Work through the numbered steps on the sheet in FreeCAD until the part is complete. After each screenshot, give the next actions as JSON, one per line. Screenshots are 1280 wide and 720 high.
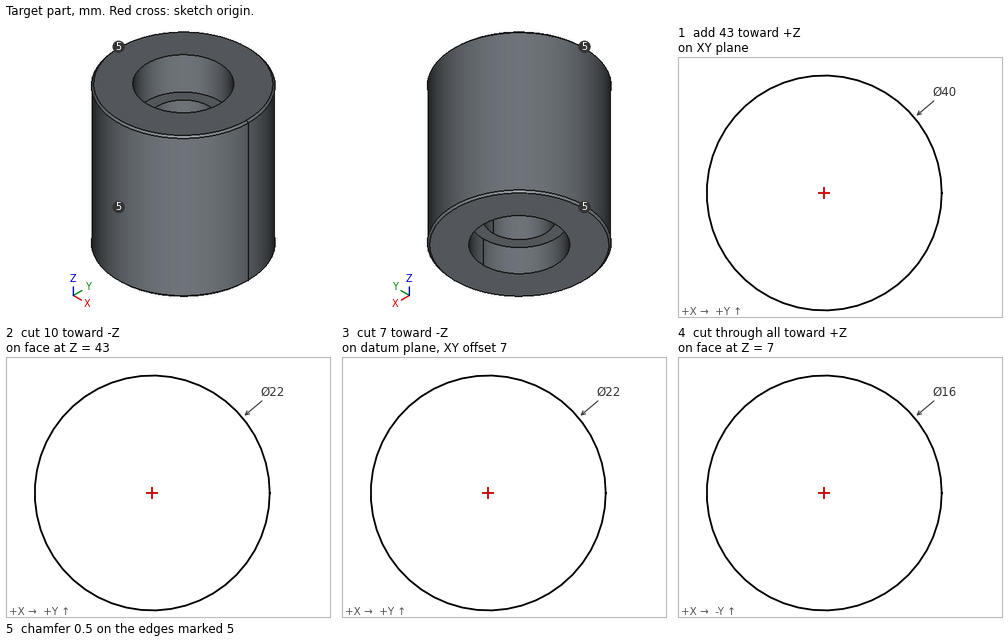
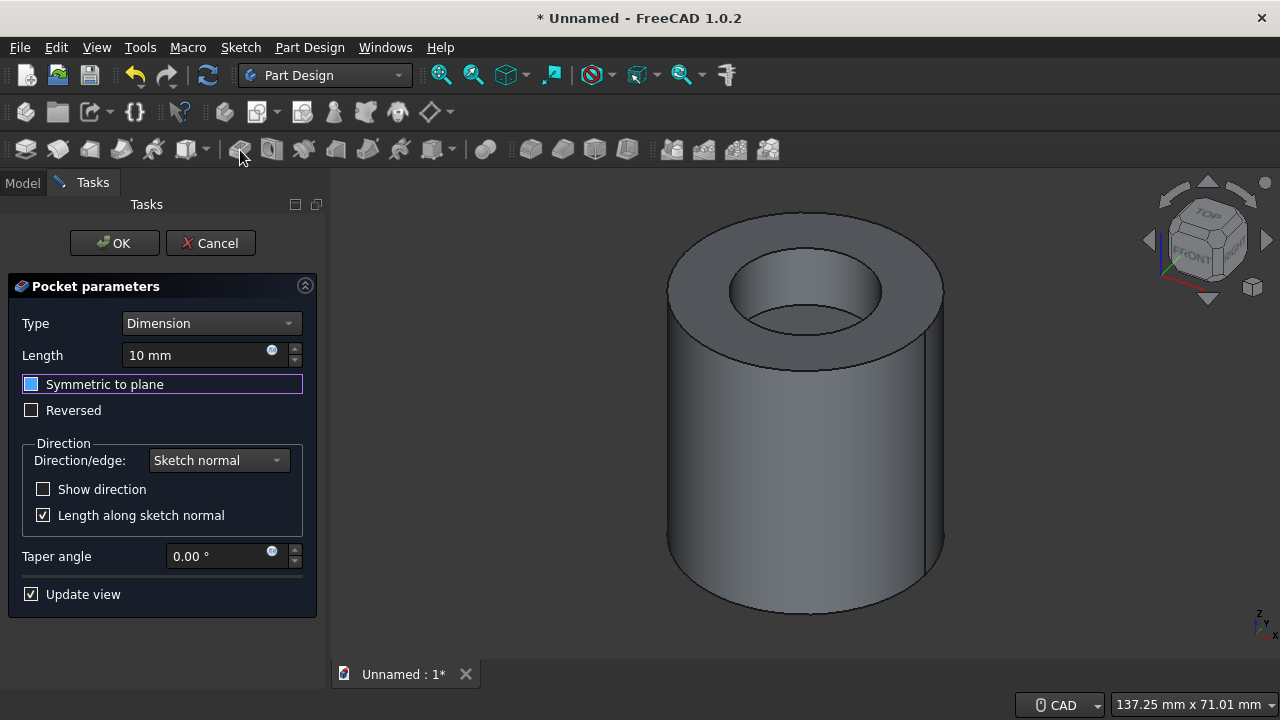
{"action": "left_click", "coordinate": [115, 243]}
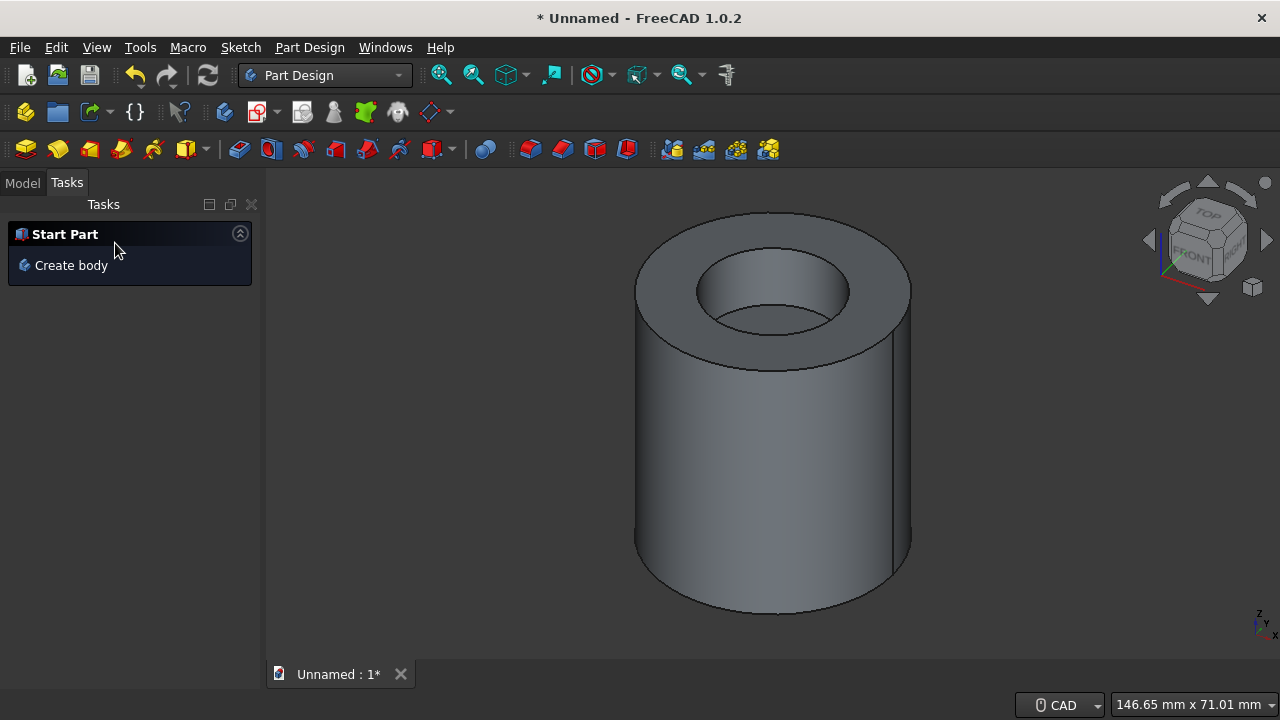
{"action": "left_click", "coordinate": [23, 182]}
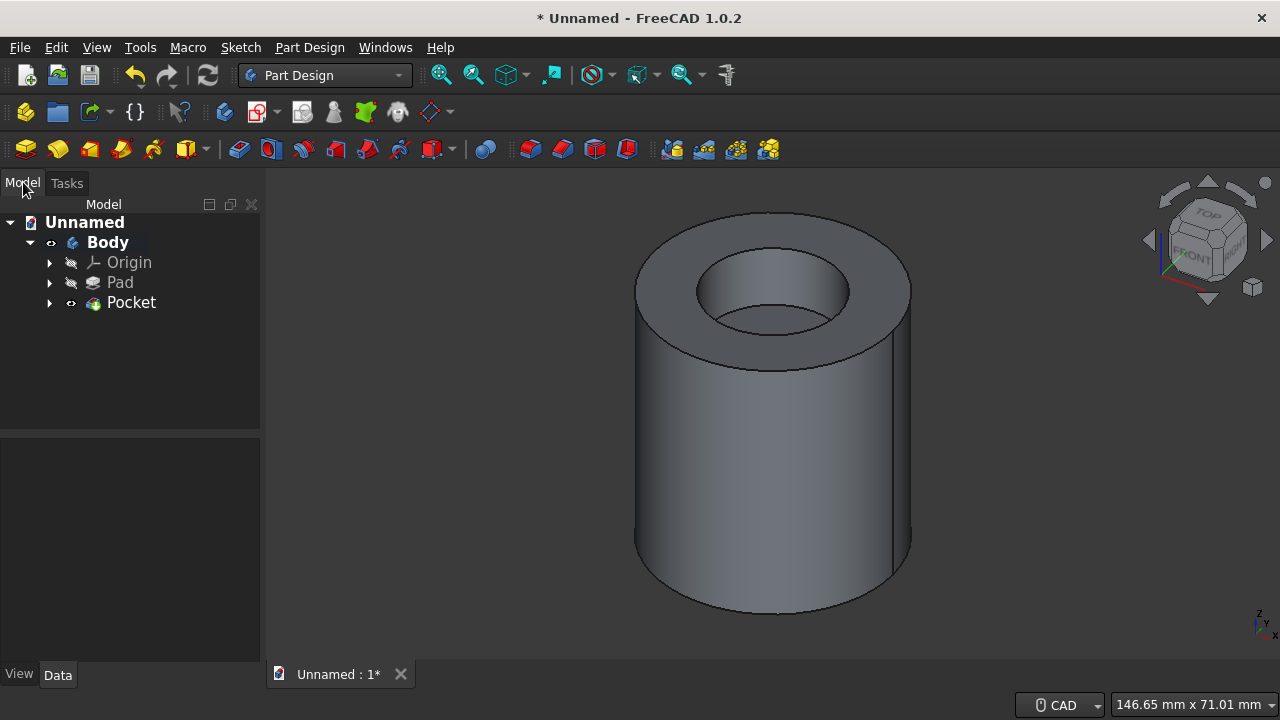
{"action": "left_click", "coordinate": [50, 263]}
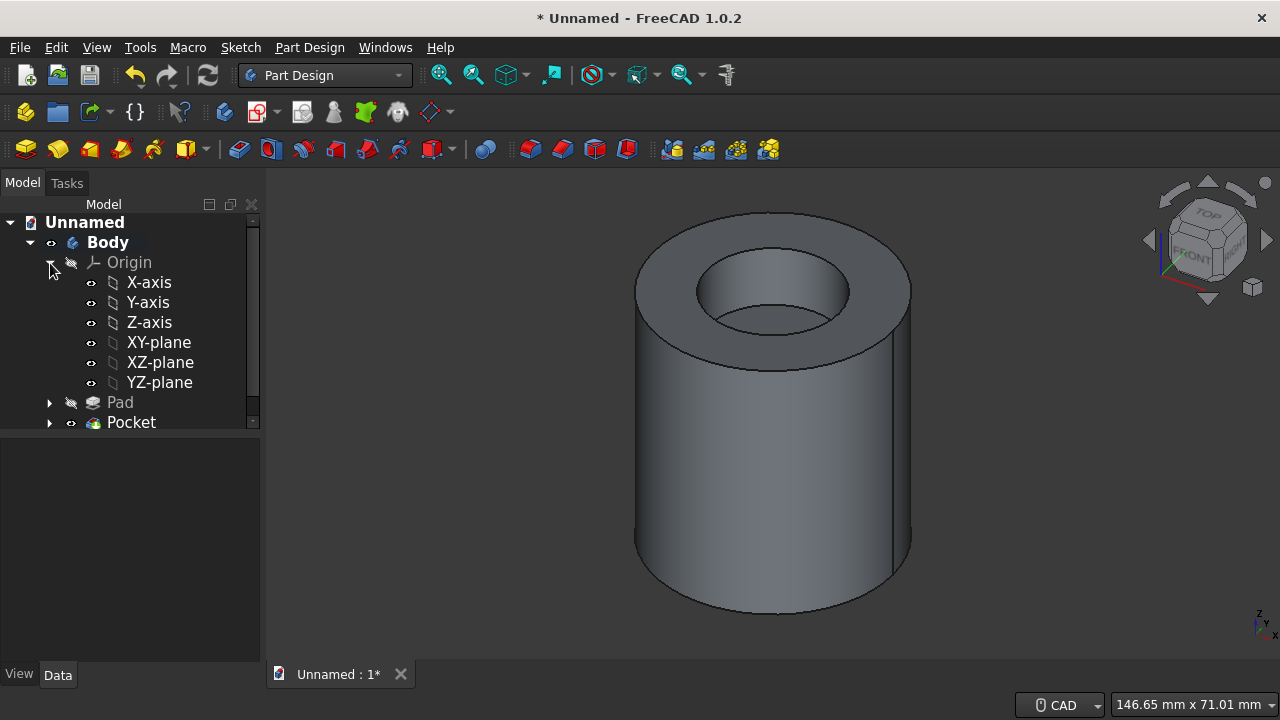
{"action": "left_click", "coordinate": [136, 343]}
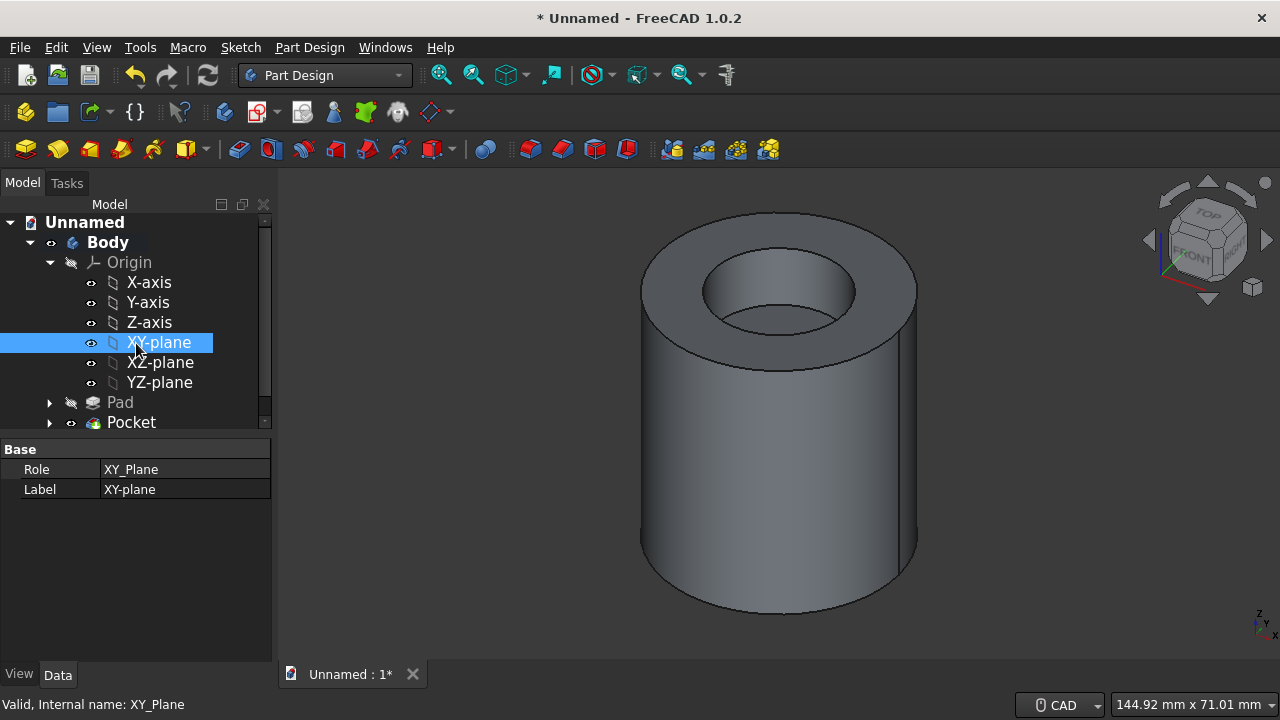
{"action": "left_click", "coordinate": [430, 112]}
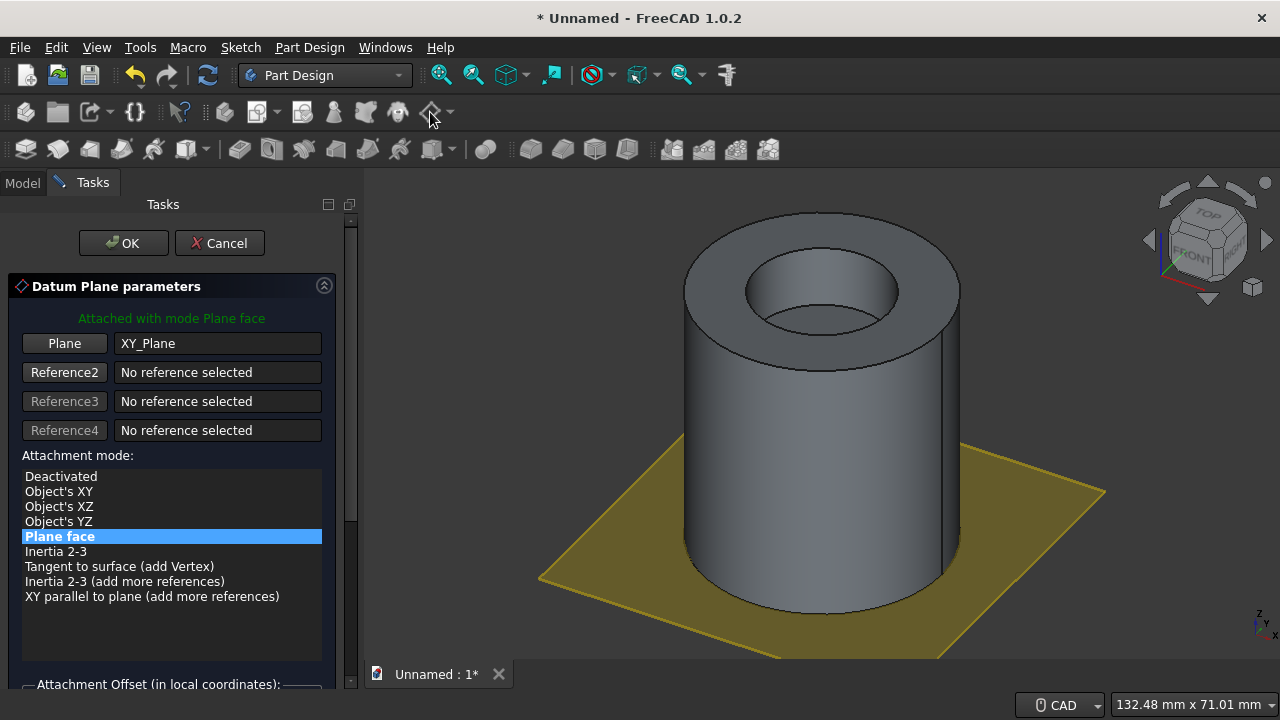
{"action": "scroll", "coordinate": [351, 451], "scroll_direction": "down", "scroll_amount": 3}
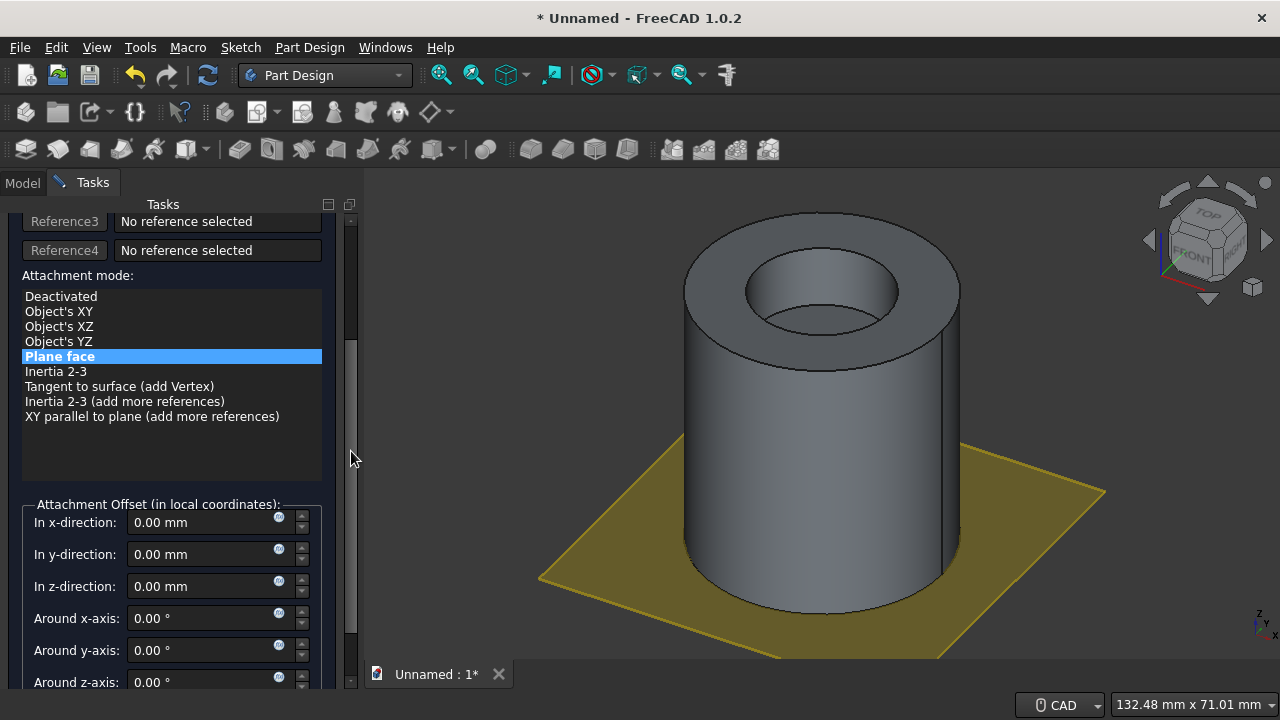
{"action": "triple_click", "coordinate": [210, 586]}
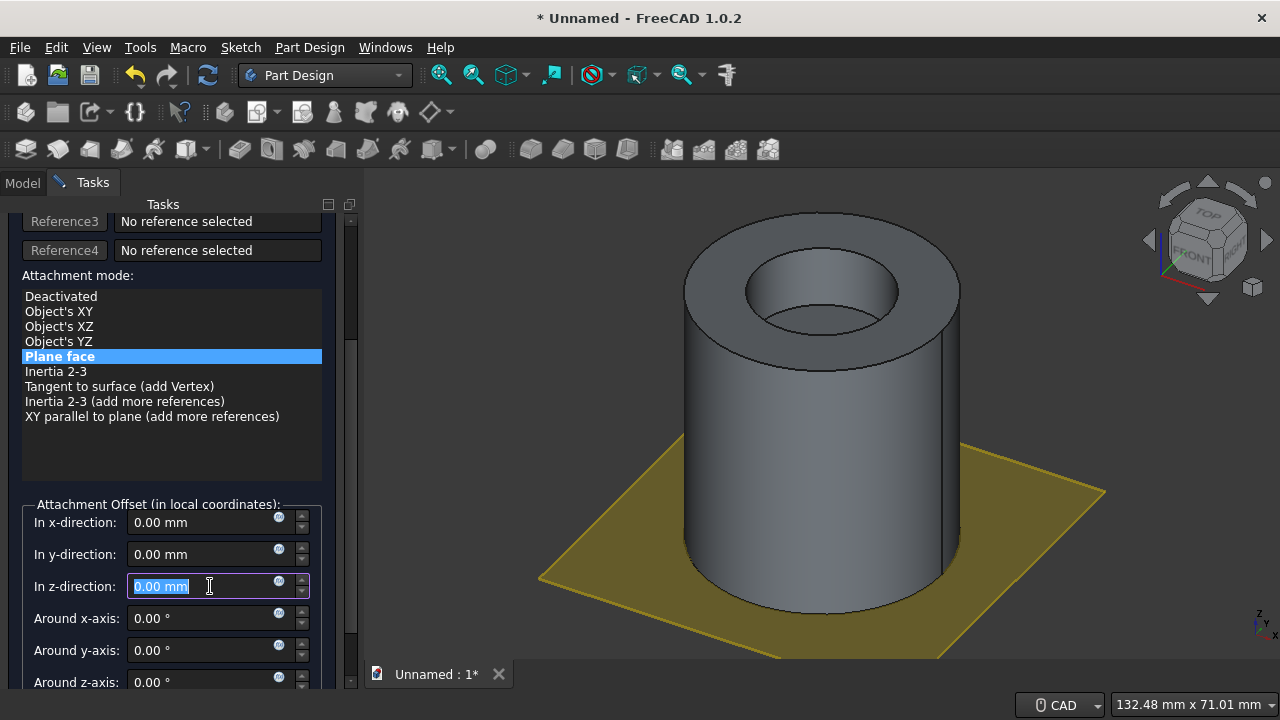
{"action": "type", "text": "7"}
{"action": "key", "text": "Tab"}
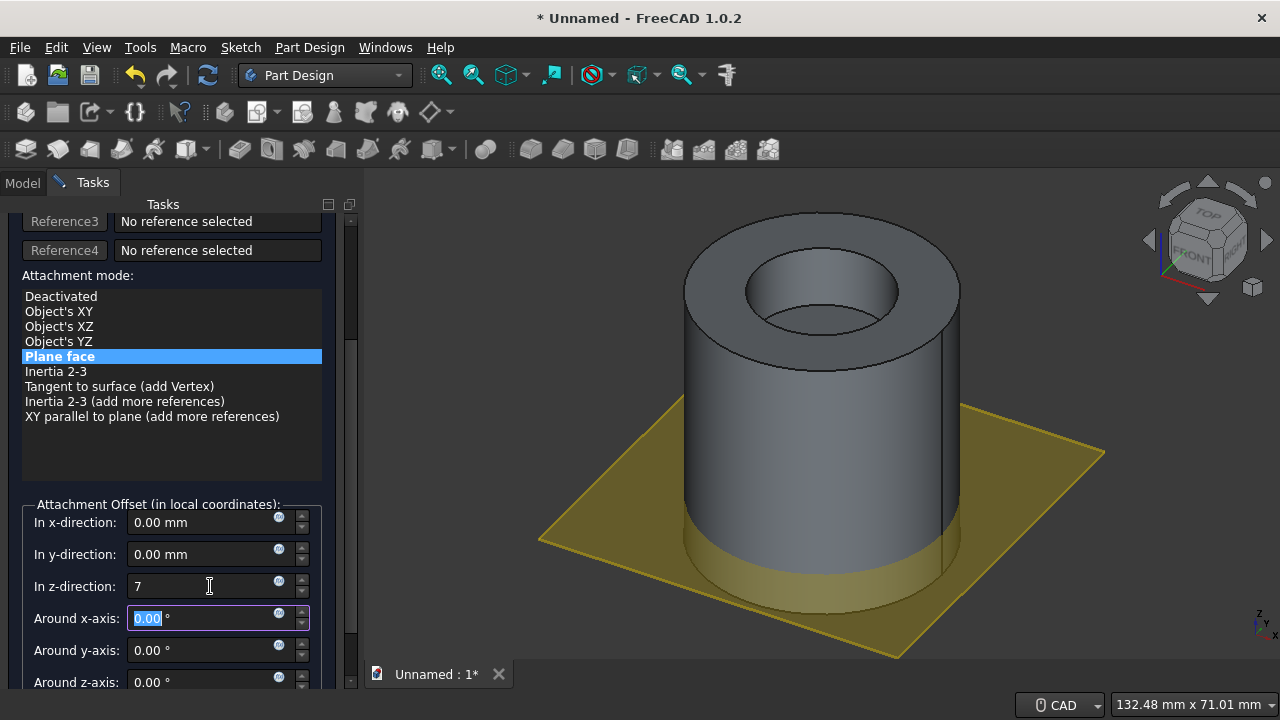
{"action": "scroll", "coordinate": [351, 451], "scroll_direction": "up", "scroll_amount": 4}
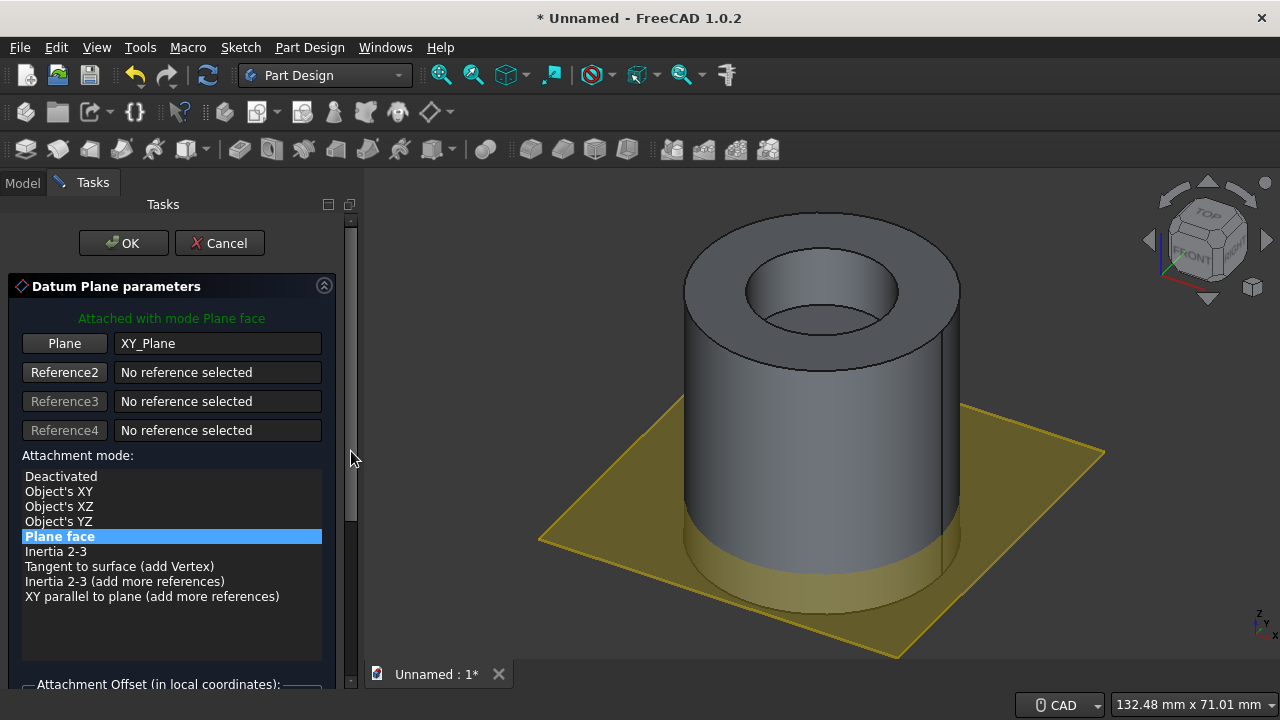
{"action": "left_click", "coordinate": [124, 243]}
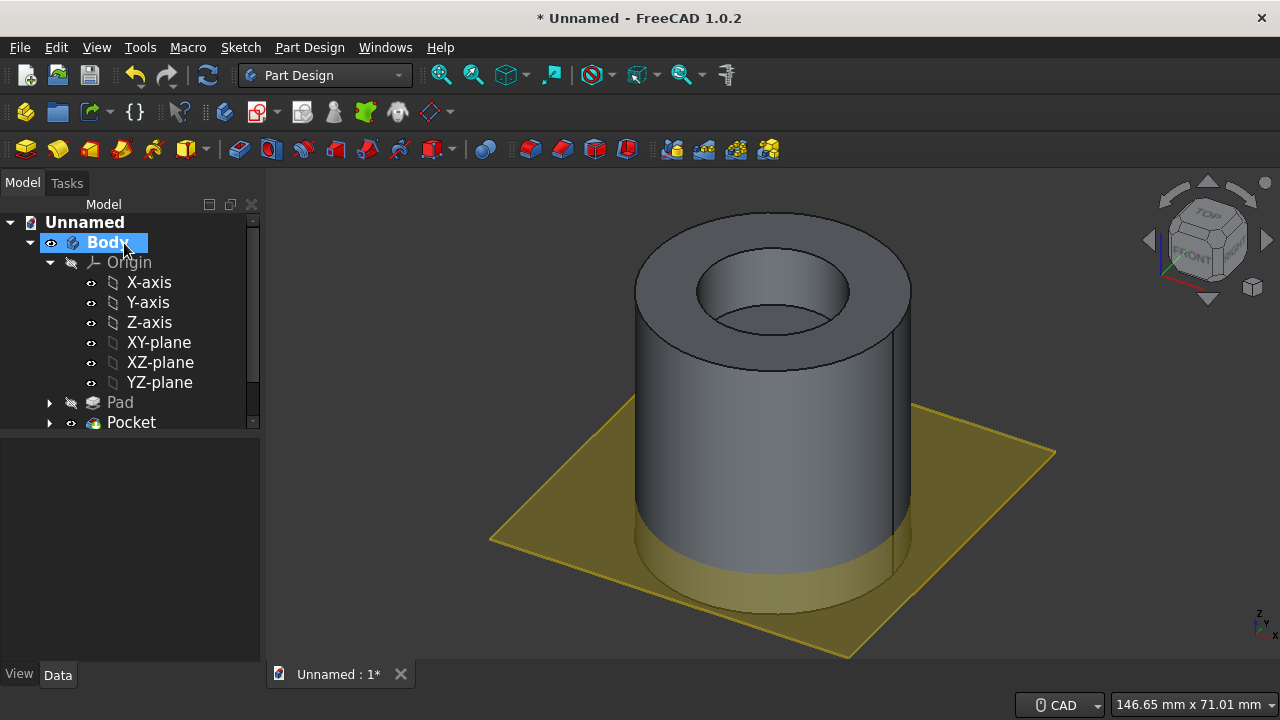
{"action": "scroll", "coordinate": [100, 318], "scroll_direction": "down", "scroll_amount": 3}